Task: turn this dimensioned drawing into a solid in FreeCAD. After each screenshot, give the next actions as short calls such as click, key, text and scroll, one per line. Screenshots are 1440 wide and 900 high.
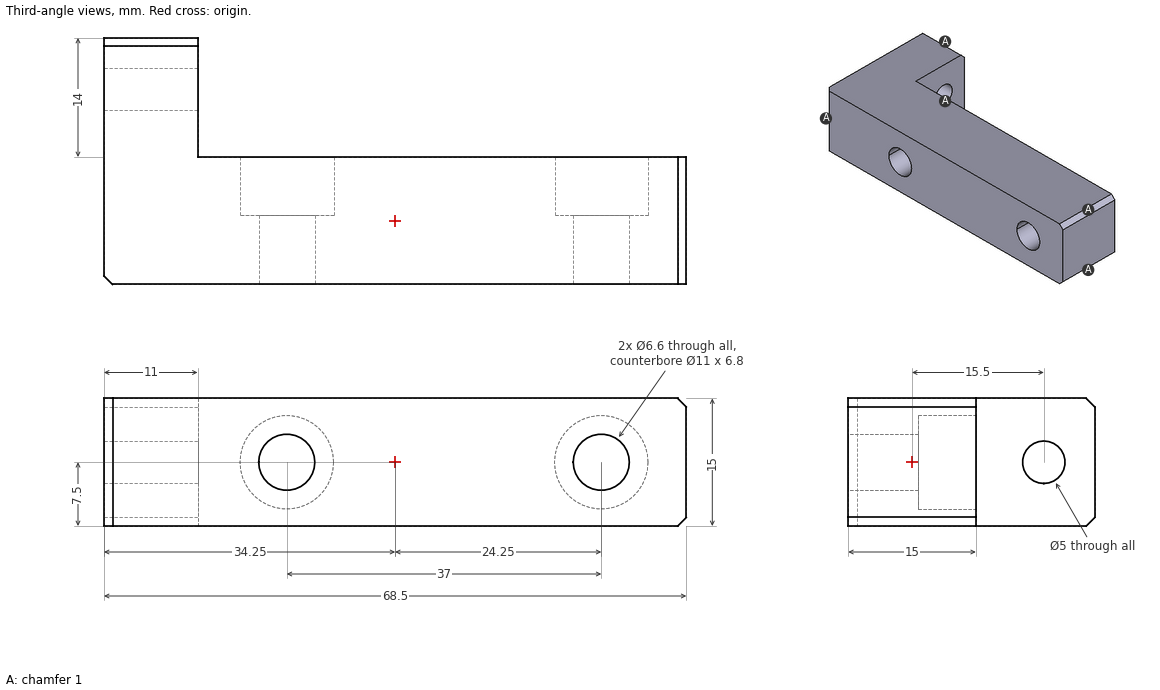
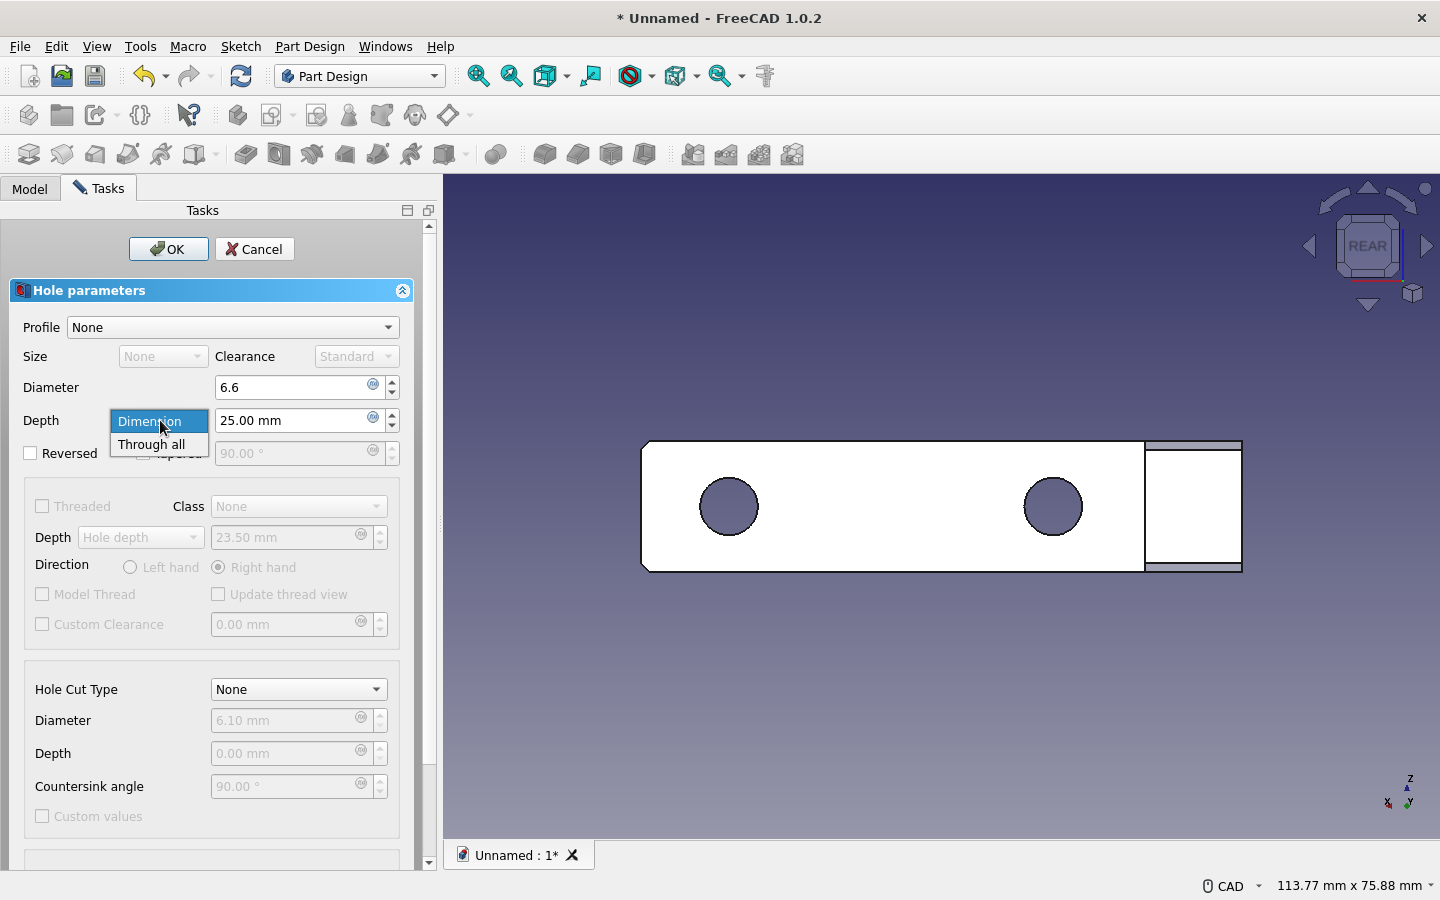
click(158, 444)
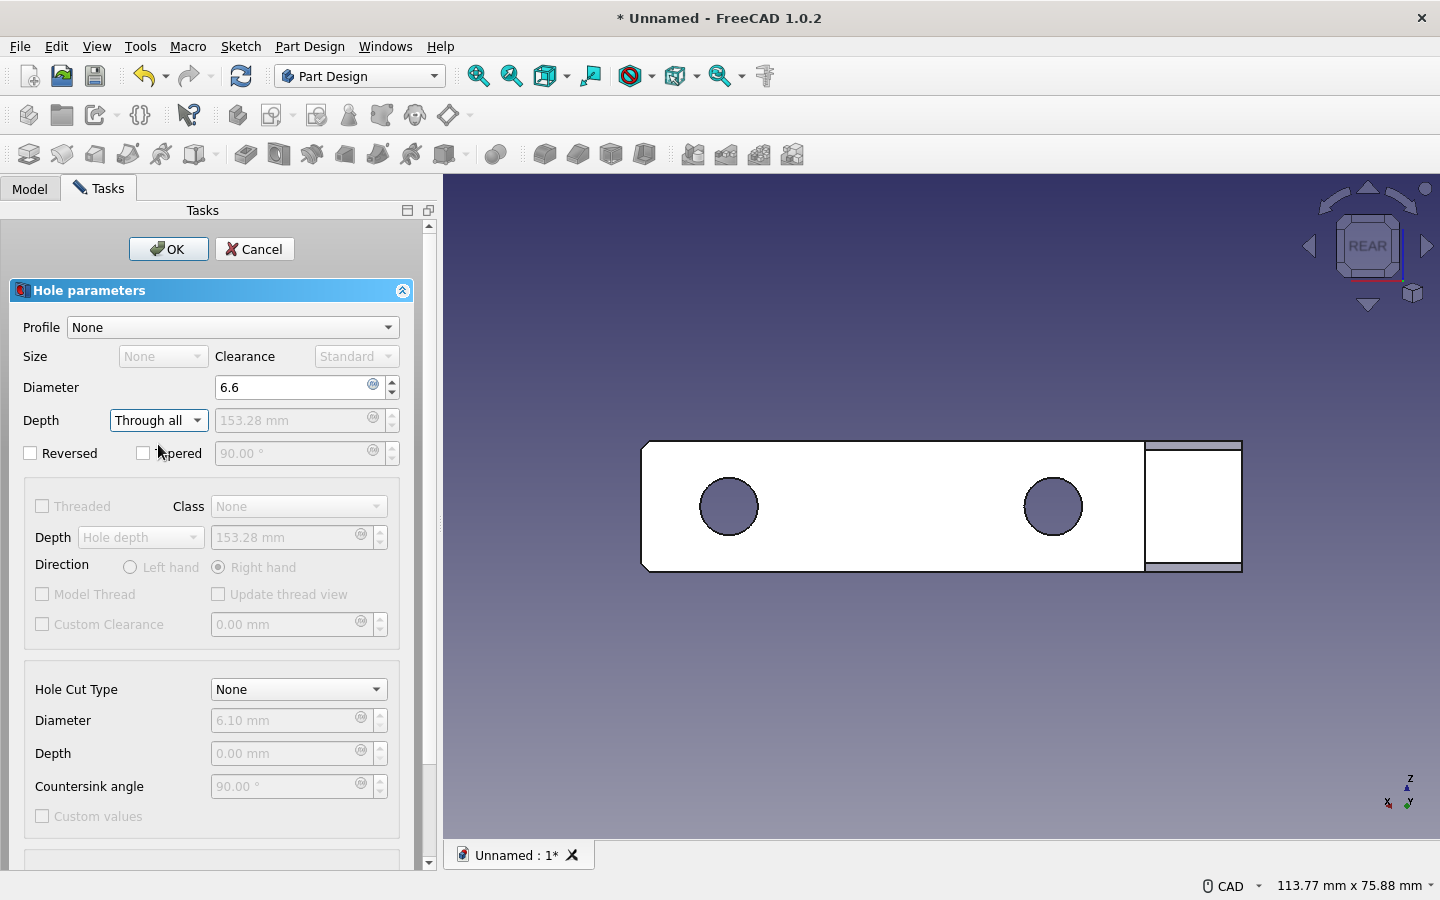
click(300, 690)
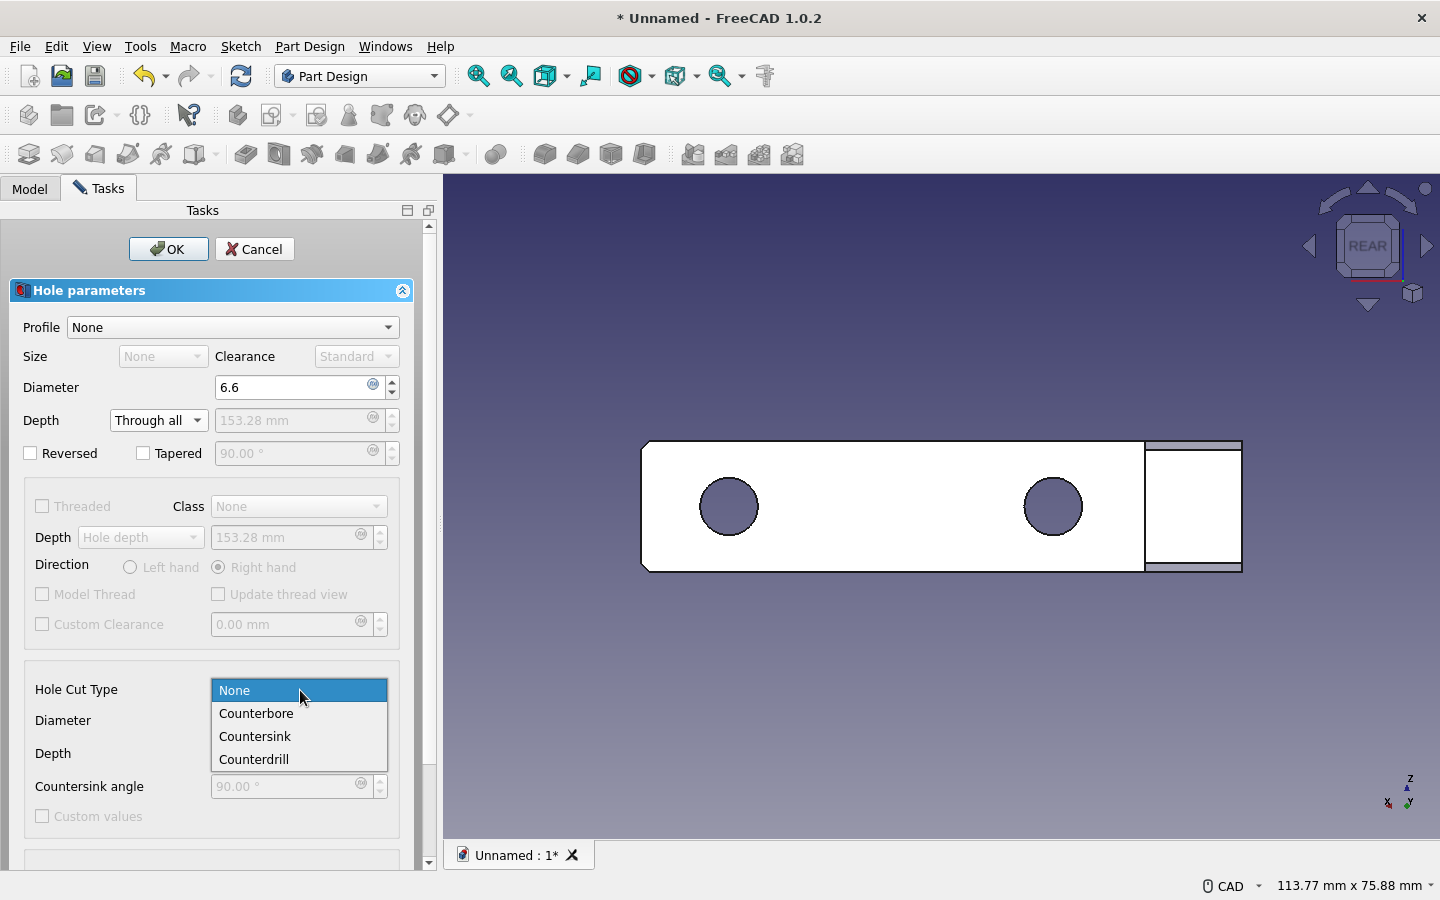
click(298, 714)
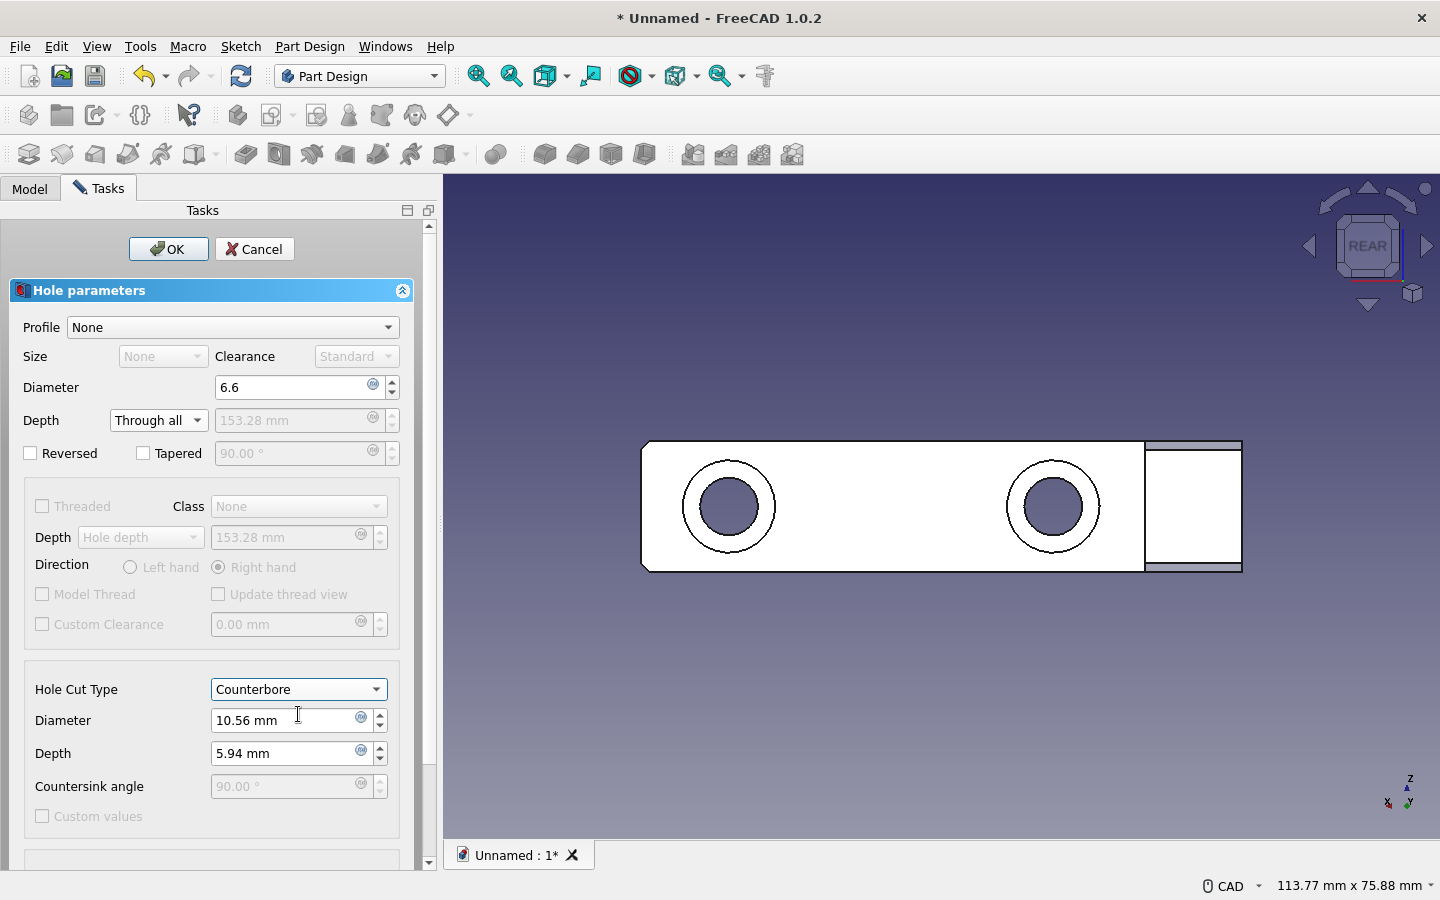
triple_click(292, 720)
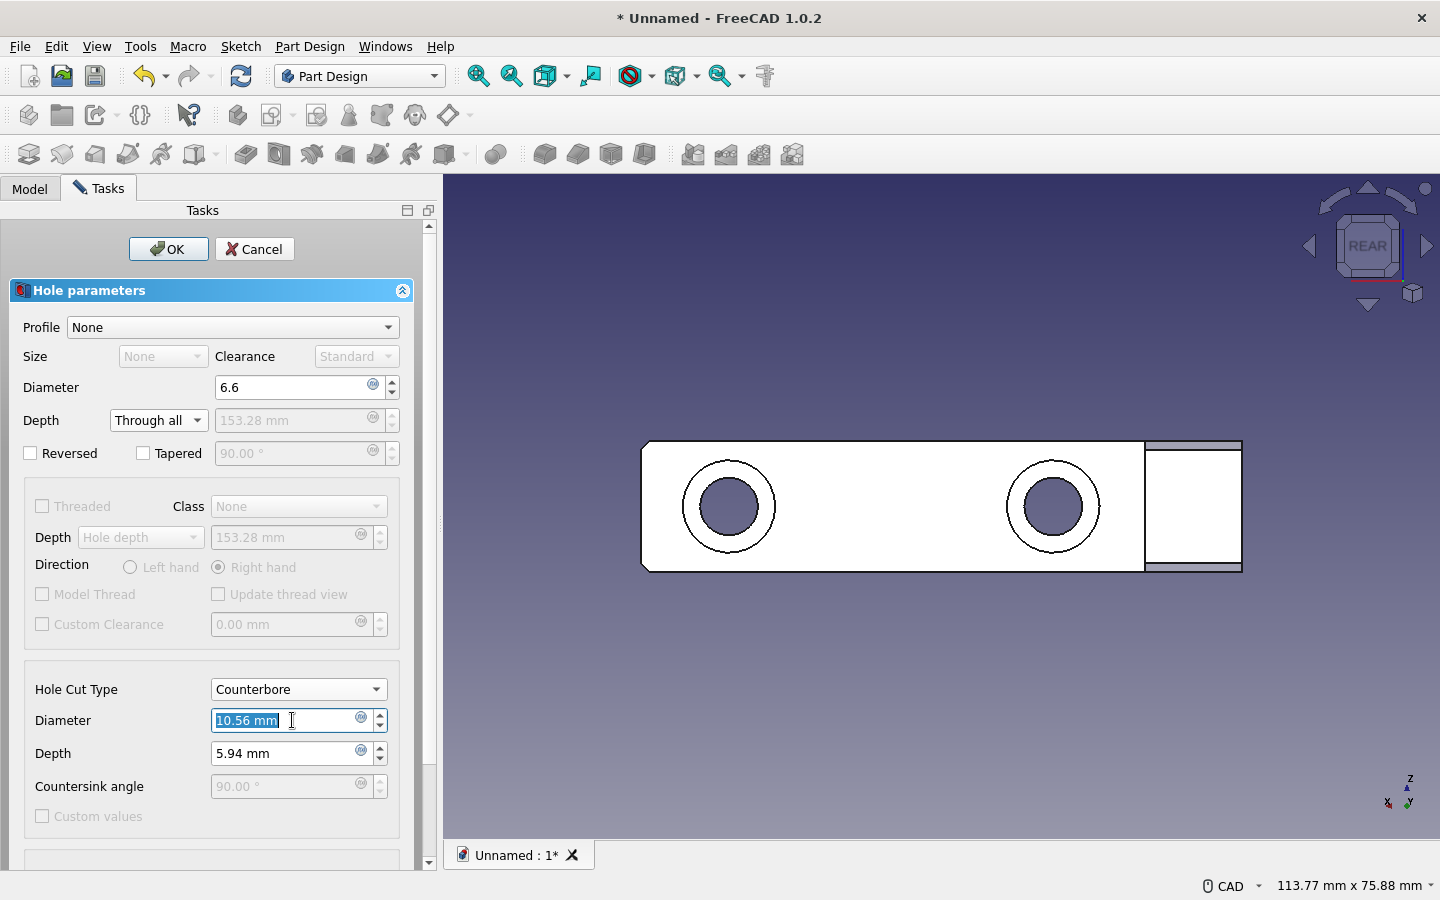
text(11)
key(Tab)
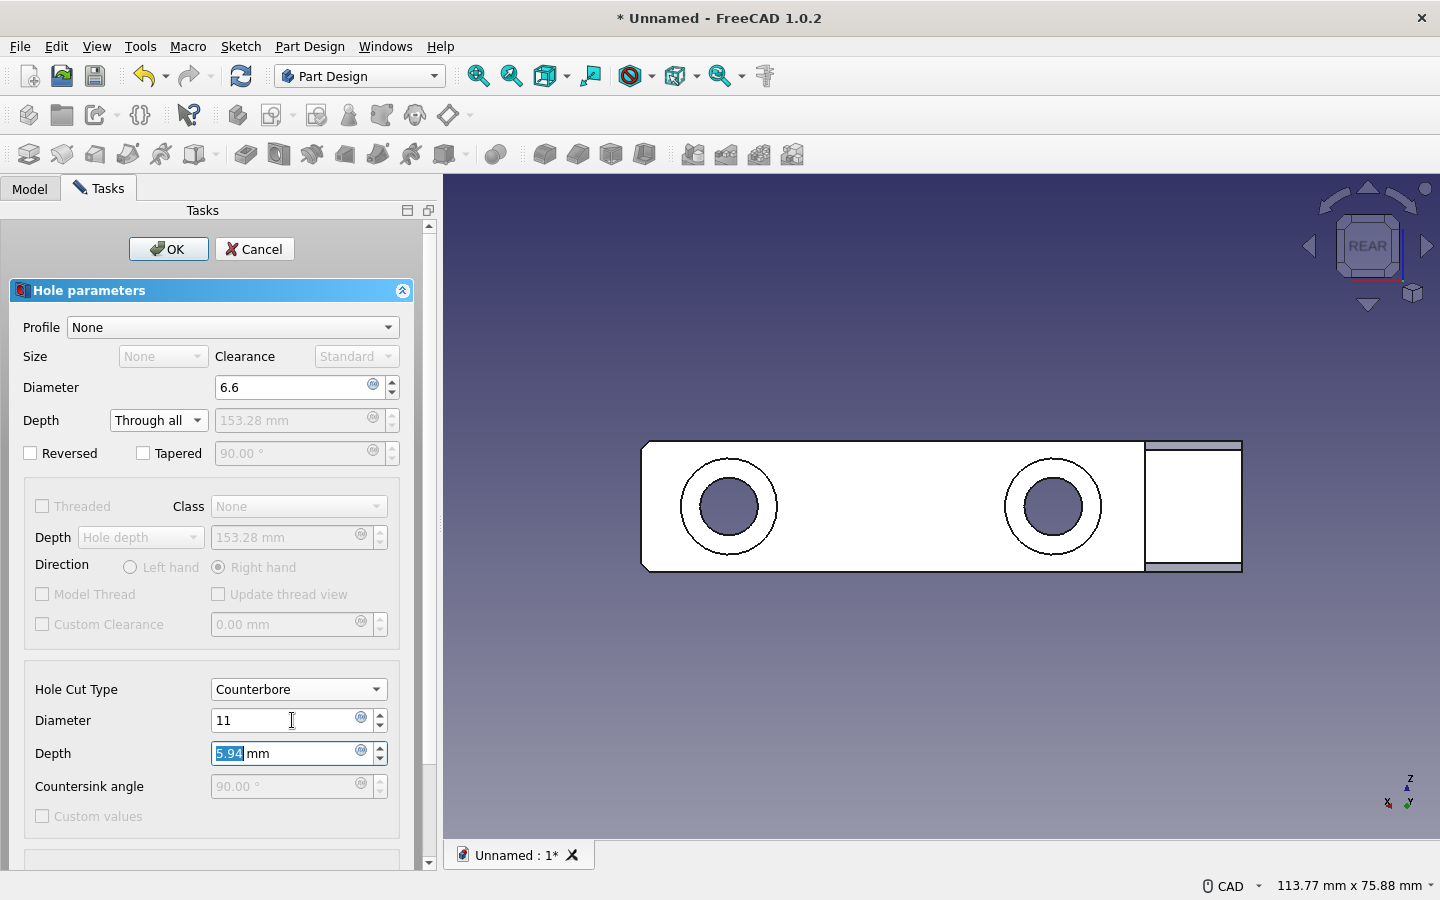
text(6.8)
key(Tab)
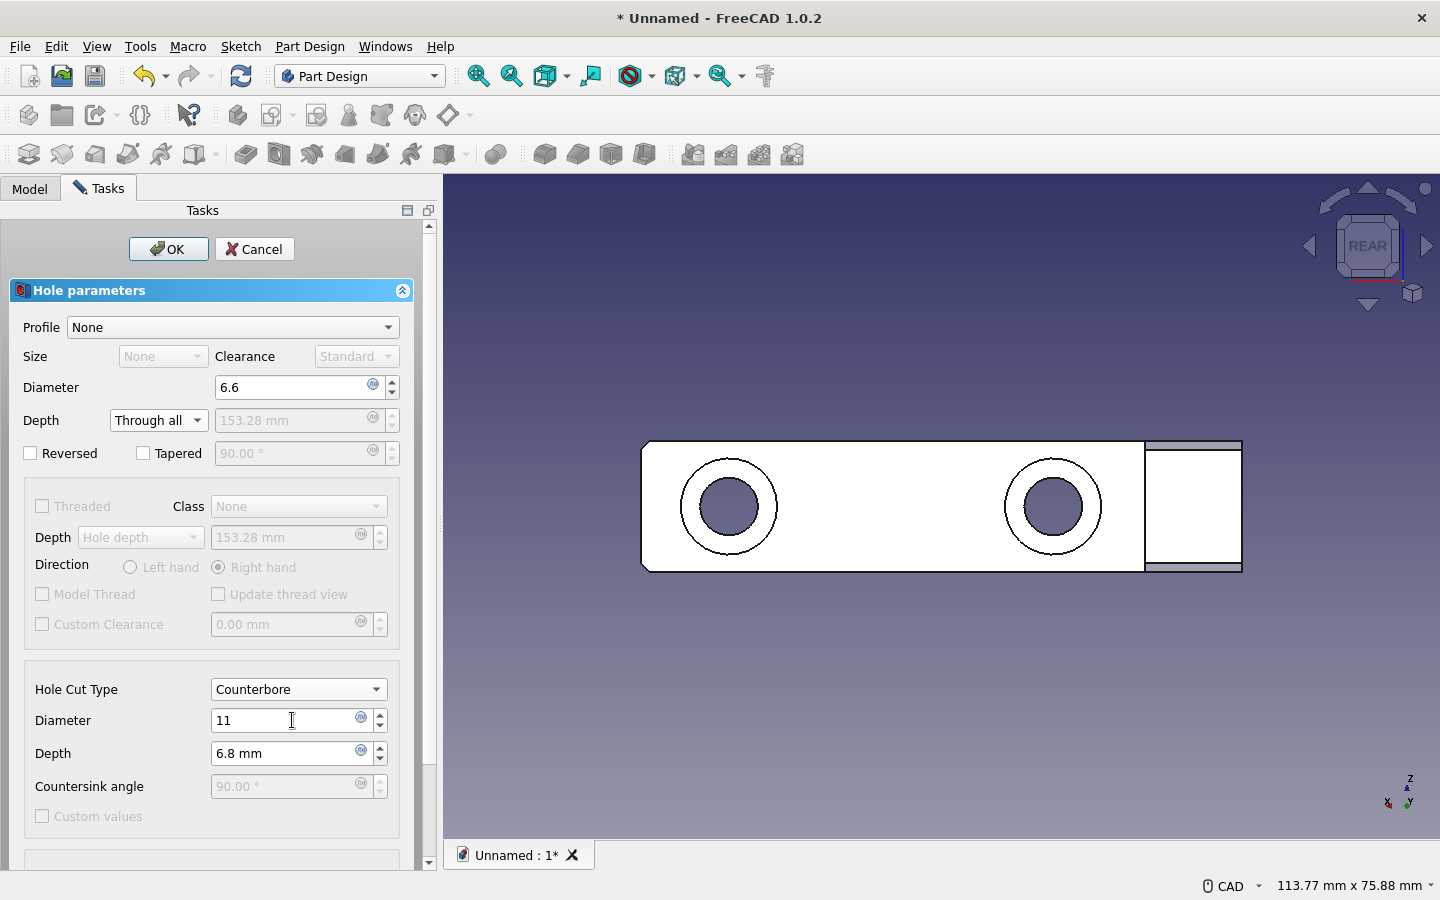
click(169, 249)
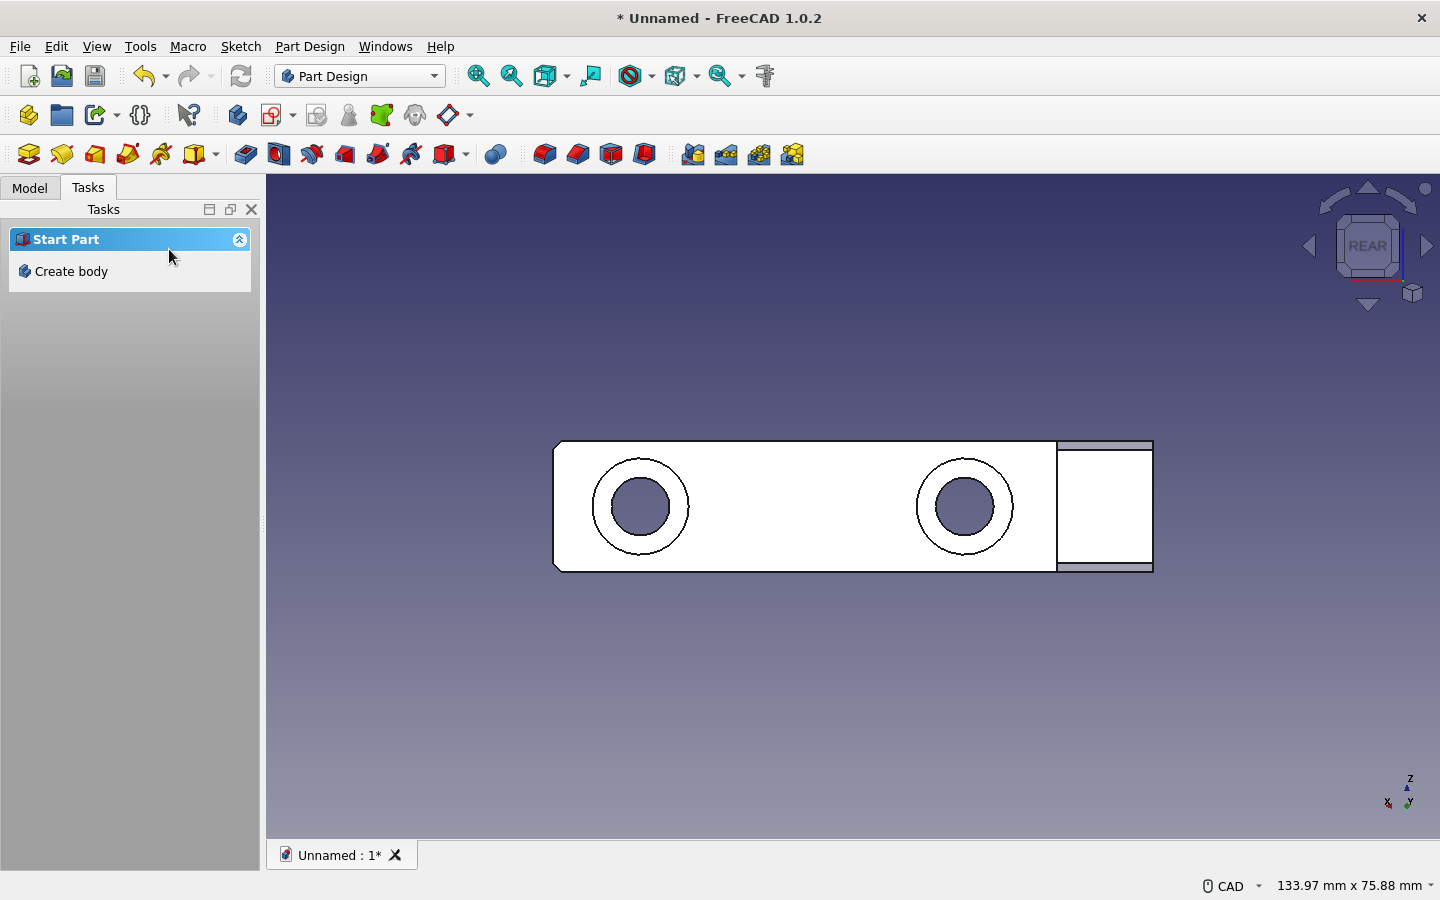
key(6)